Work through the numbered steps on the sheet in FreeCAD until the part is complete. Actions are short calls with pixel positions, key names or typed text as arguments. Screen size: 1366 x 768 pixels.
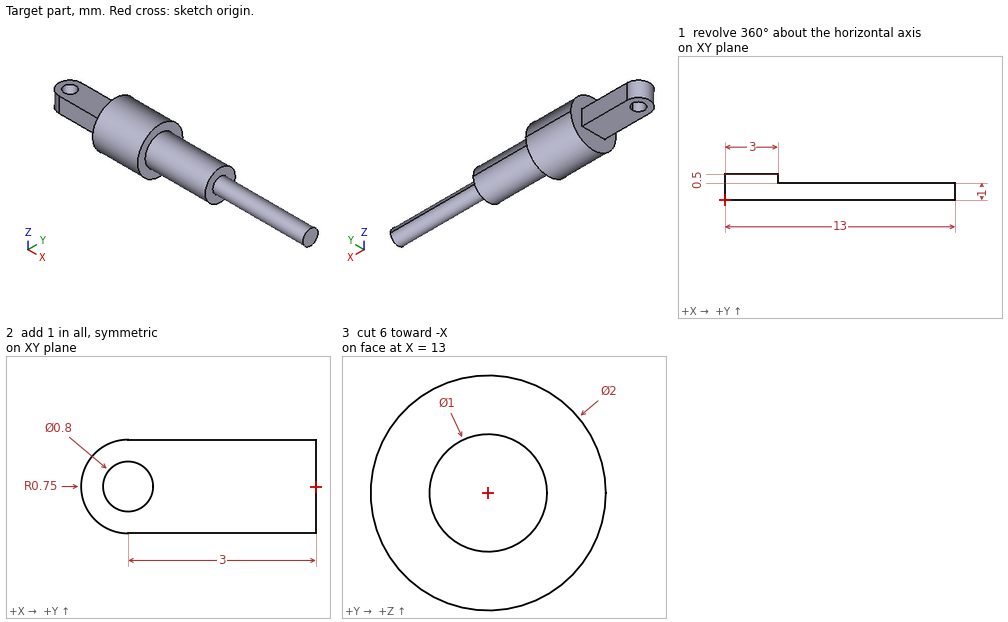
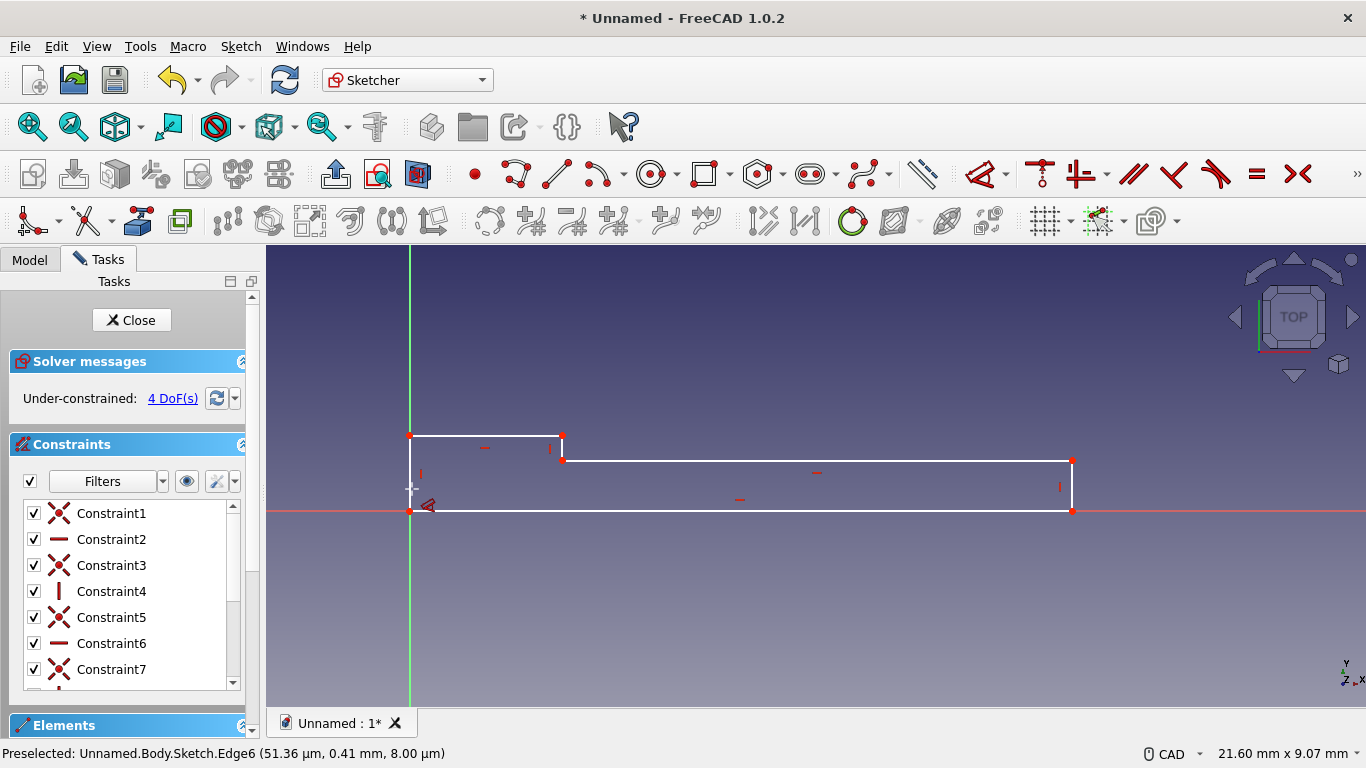
click(1072, 496)
click(1106, 486)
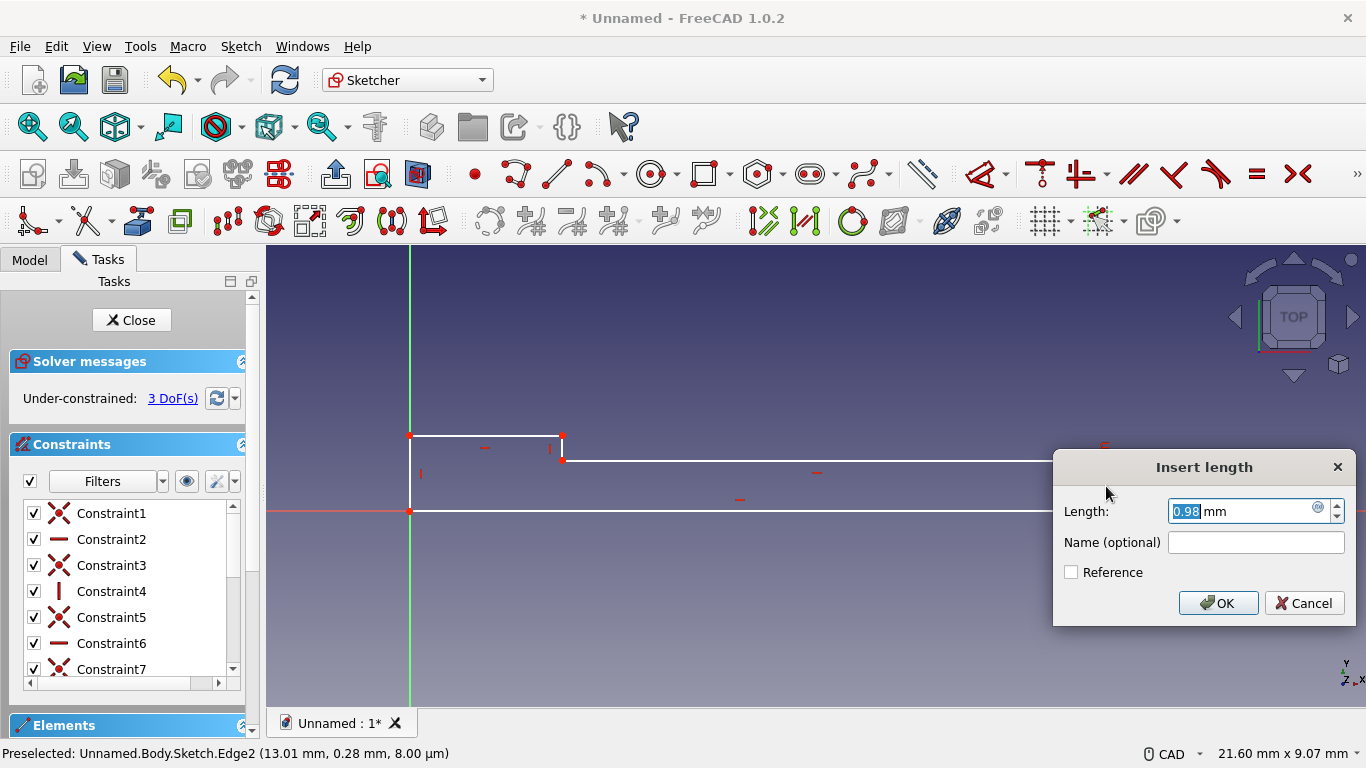
text(1)
key(Return)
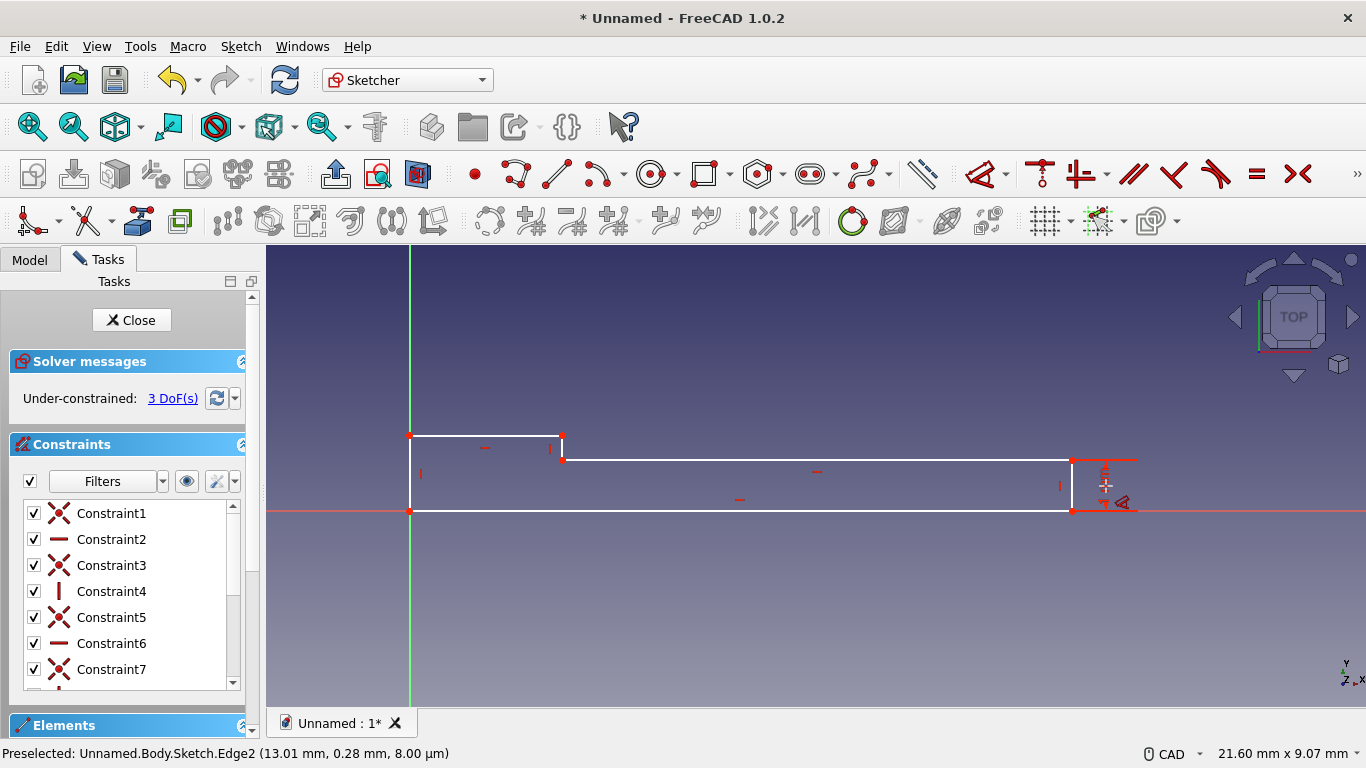
click(516, 436)
click(486, 402)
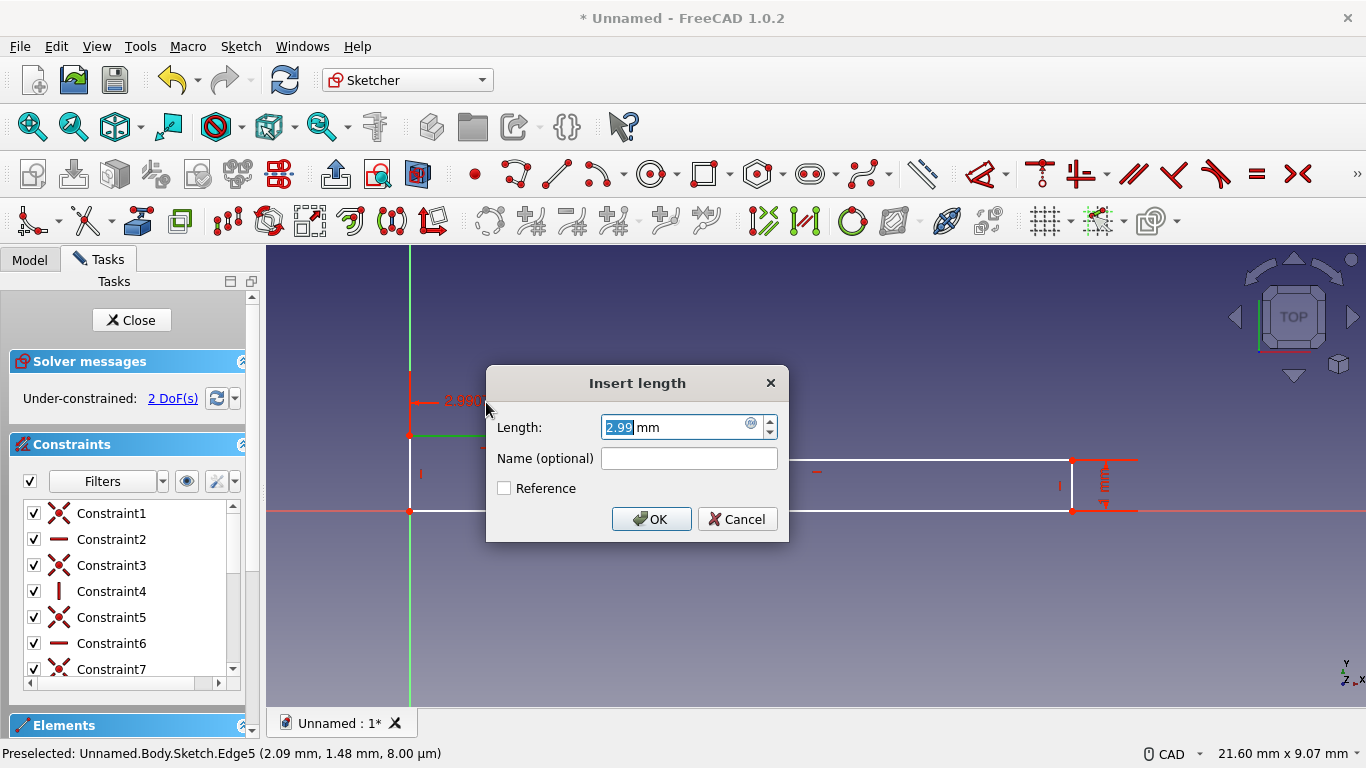
text(3)
key(Return)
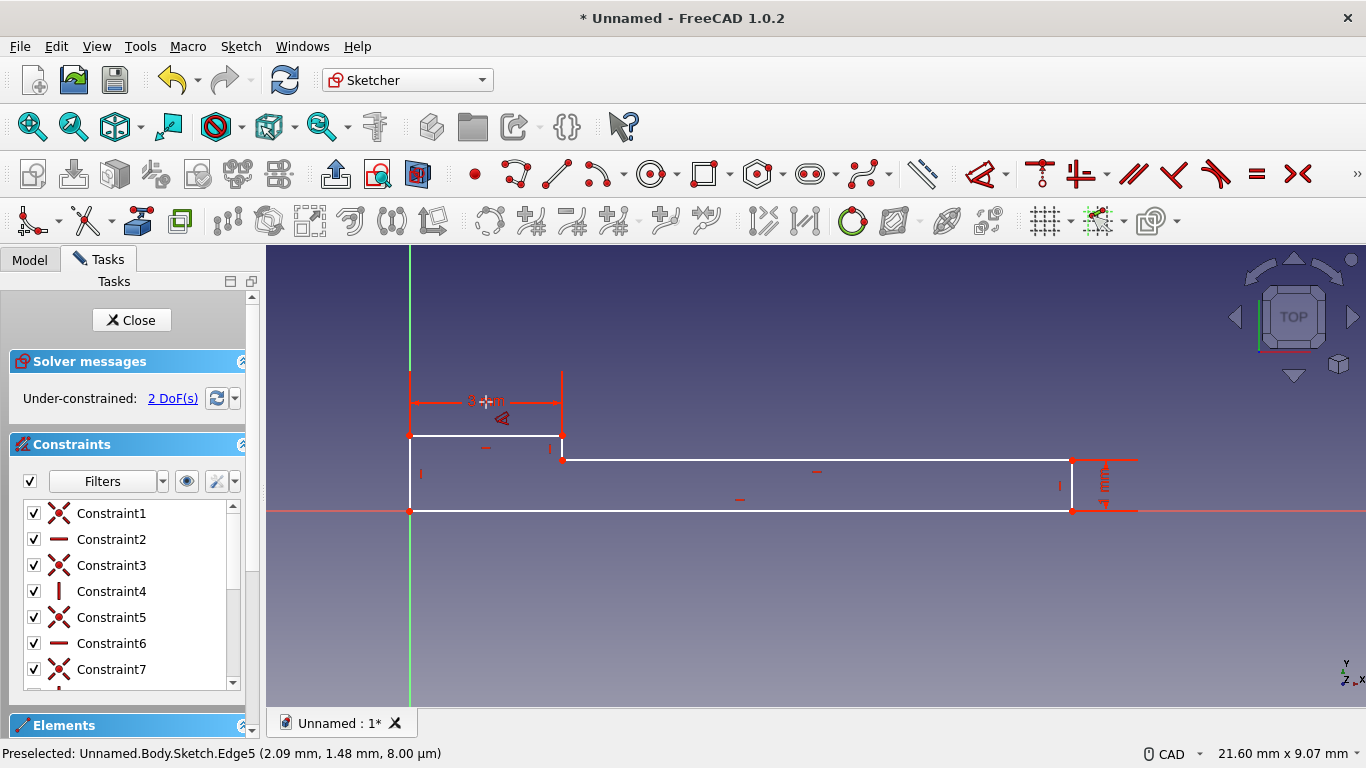
click(608, 511)
click(741, 545)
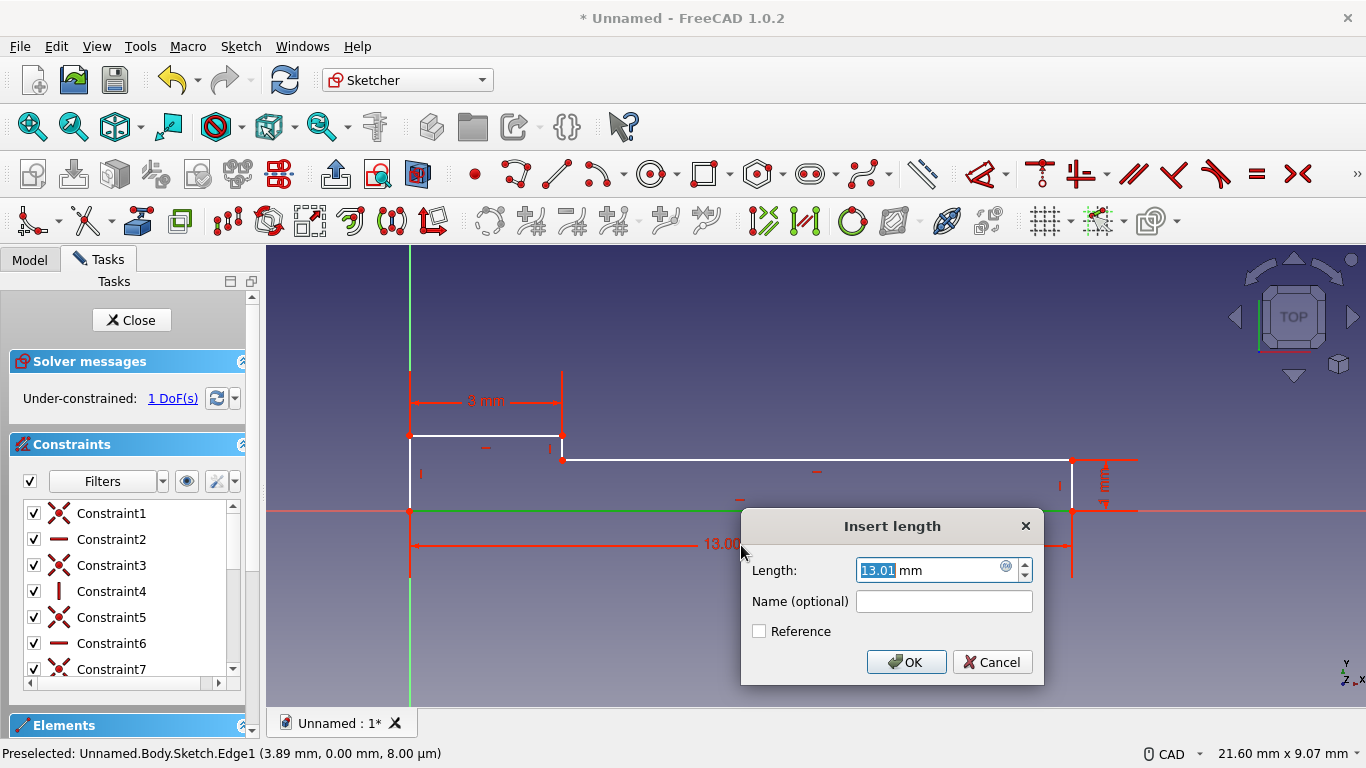
text(13)
key(Return)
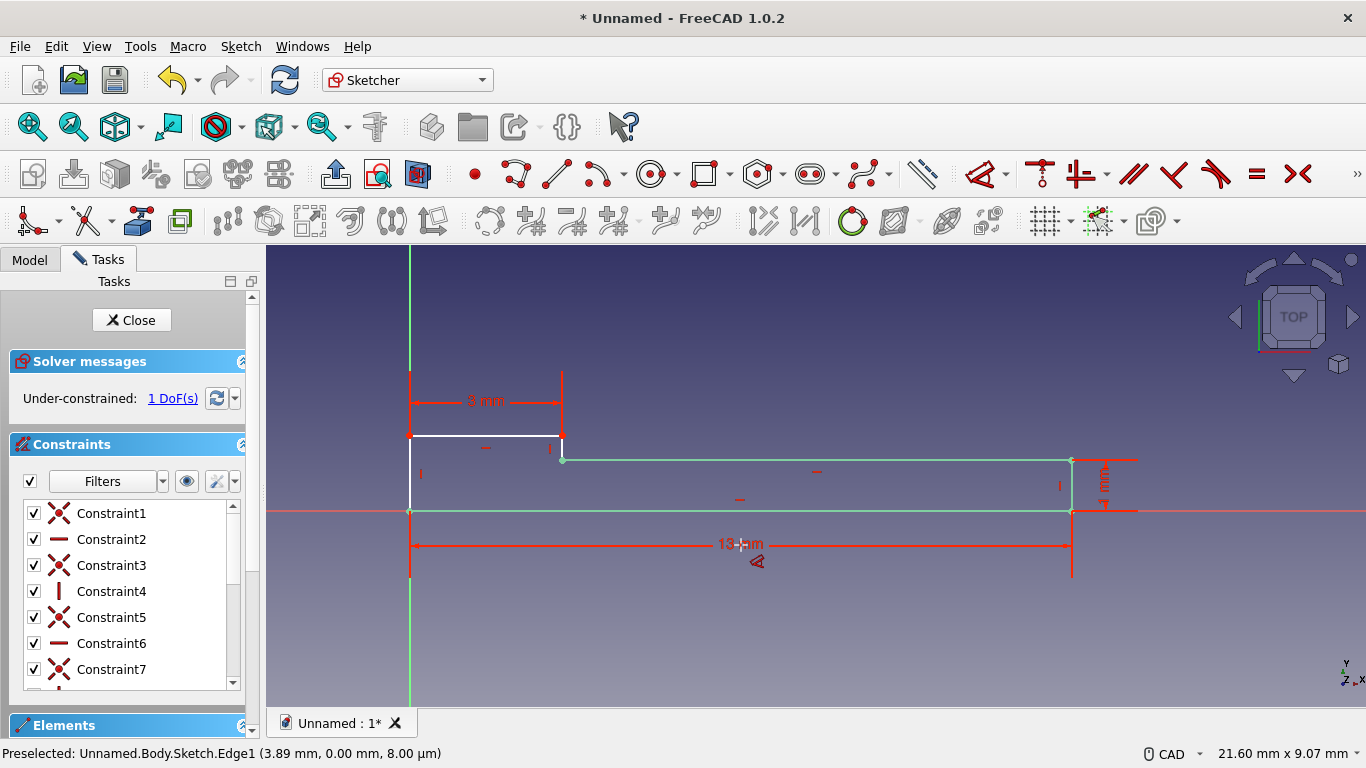
scroll(562, 451, up, 3)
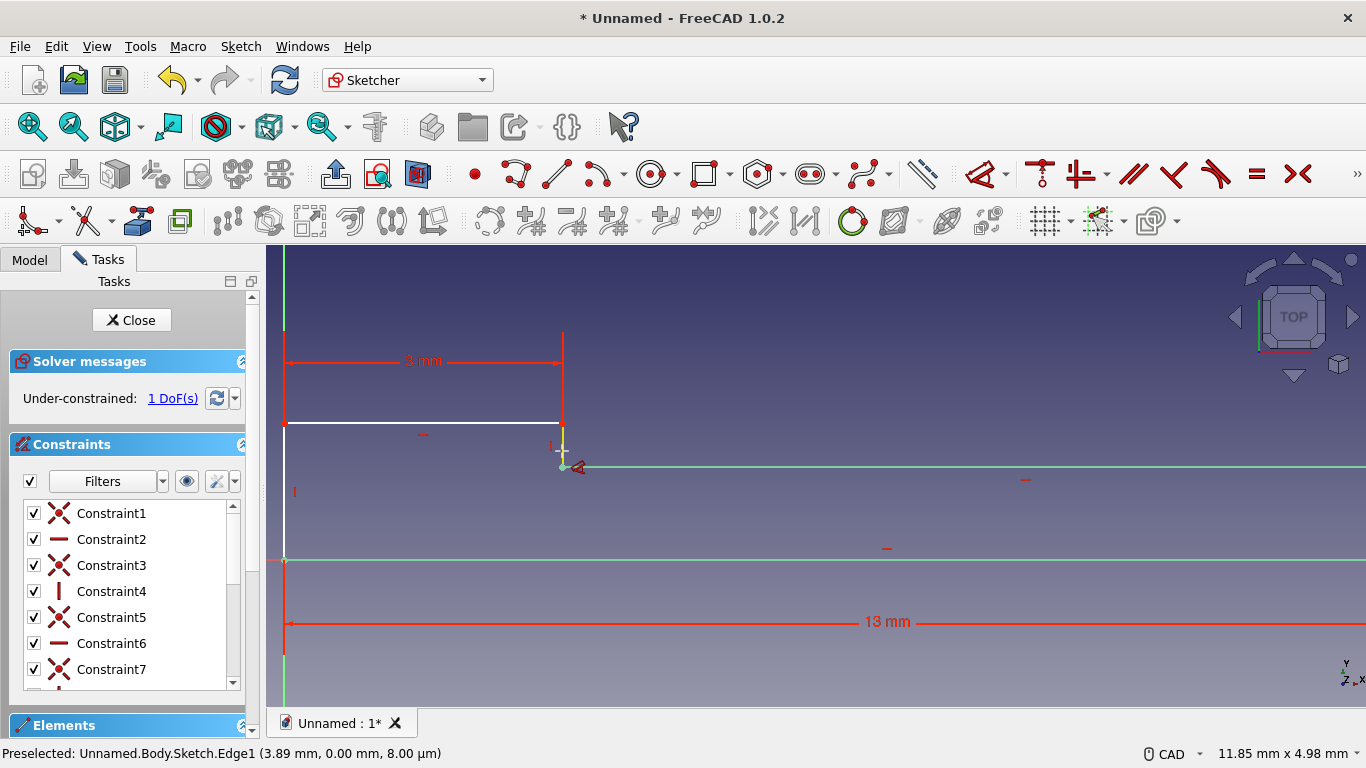
click(563, 450)
click(529, 445)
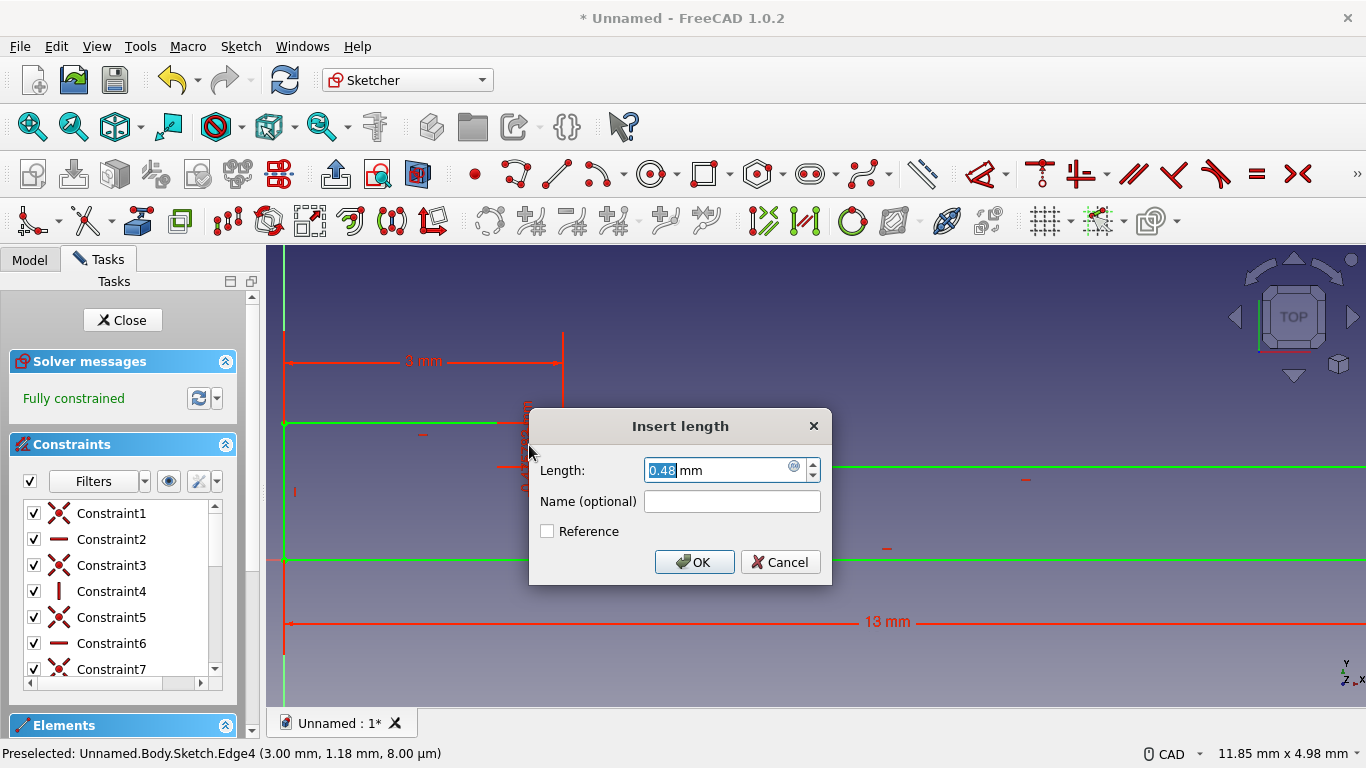
text(0.5)
key(Return)
key(Escape)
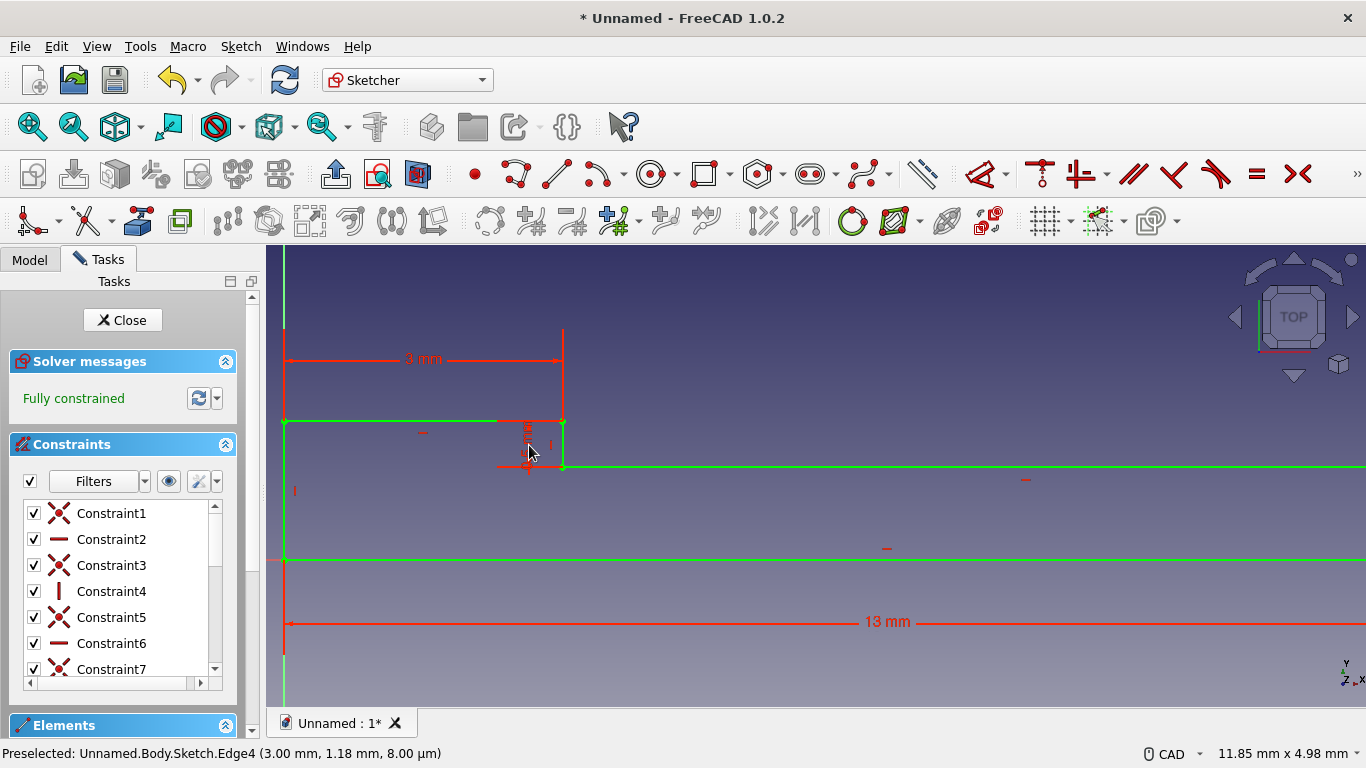
click(123, 320)